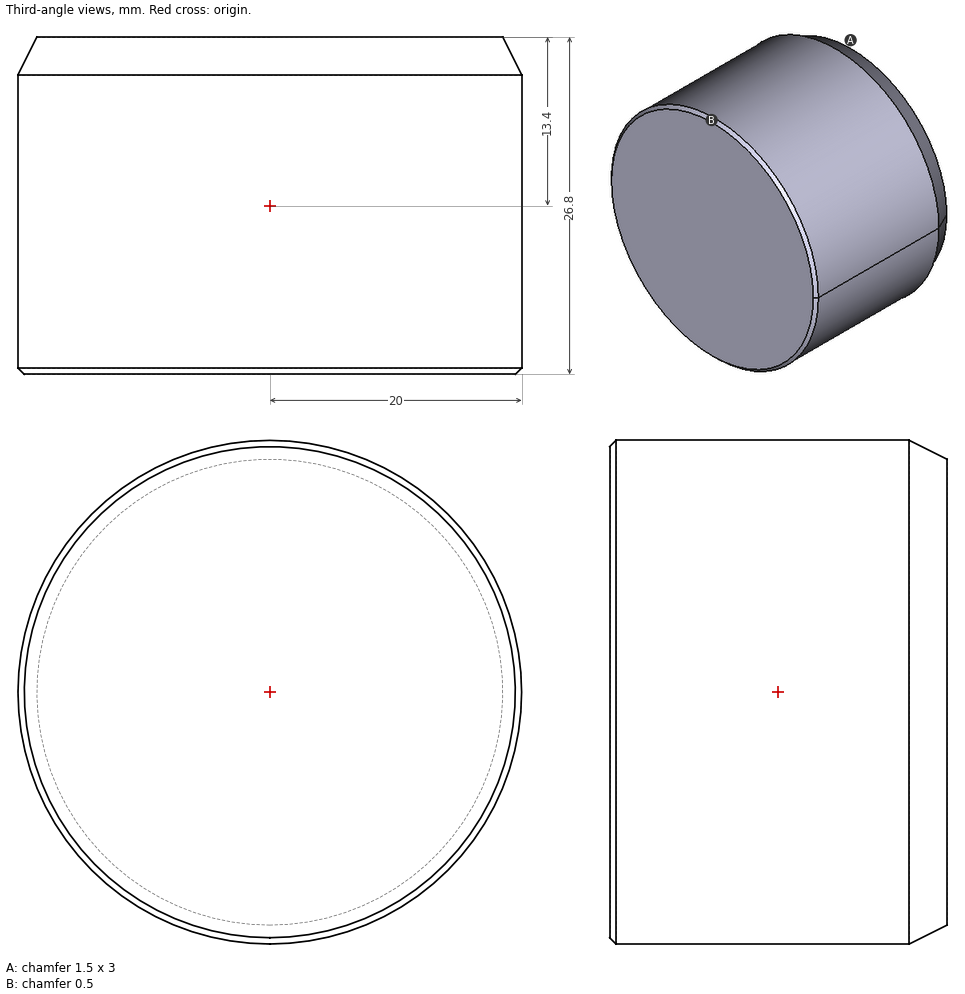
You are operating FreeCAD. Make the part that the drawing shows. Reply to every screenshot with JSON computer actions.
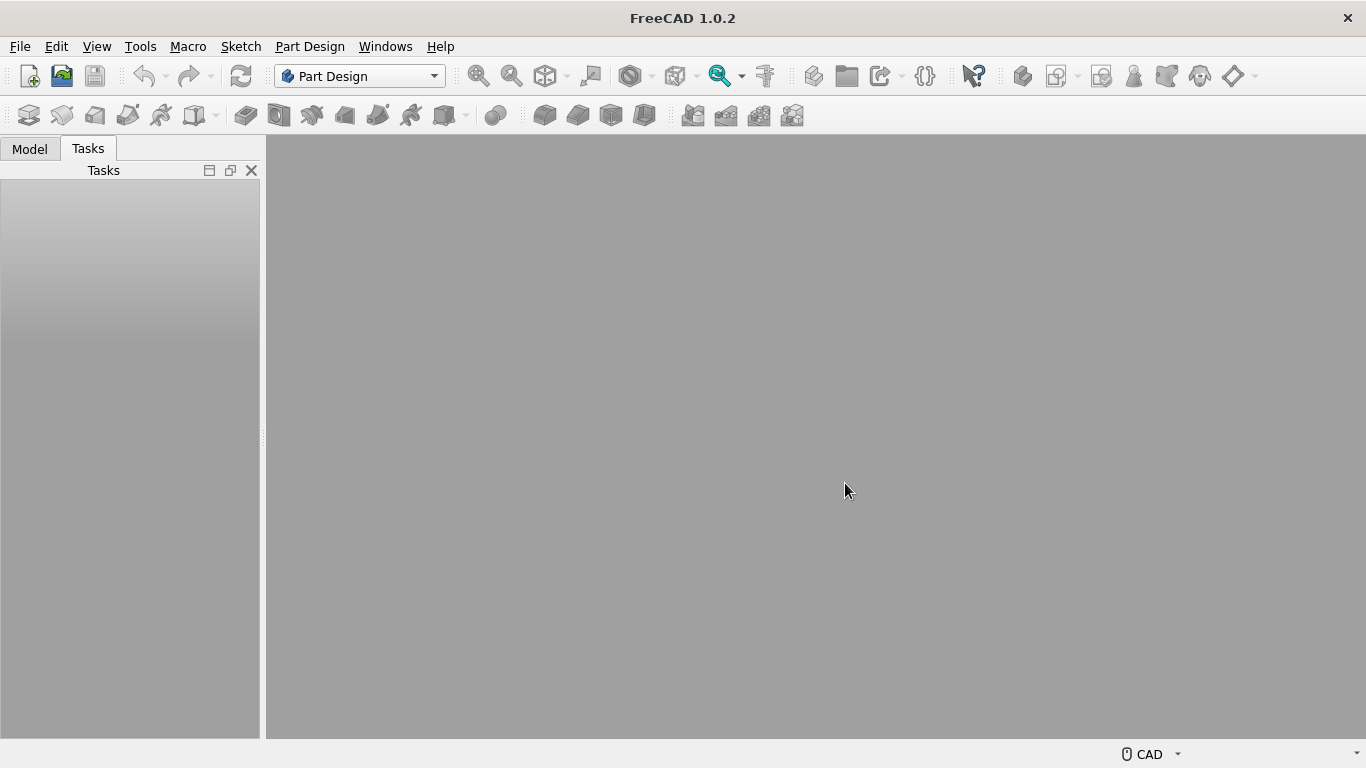
{"action": "left_click", "coordinate": [29, 76]}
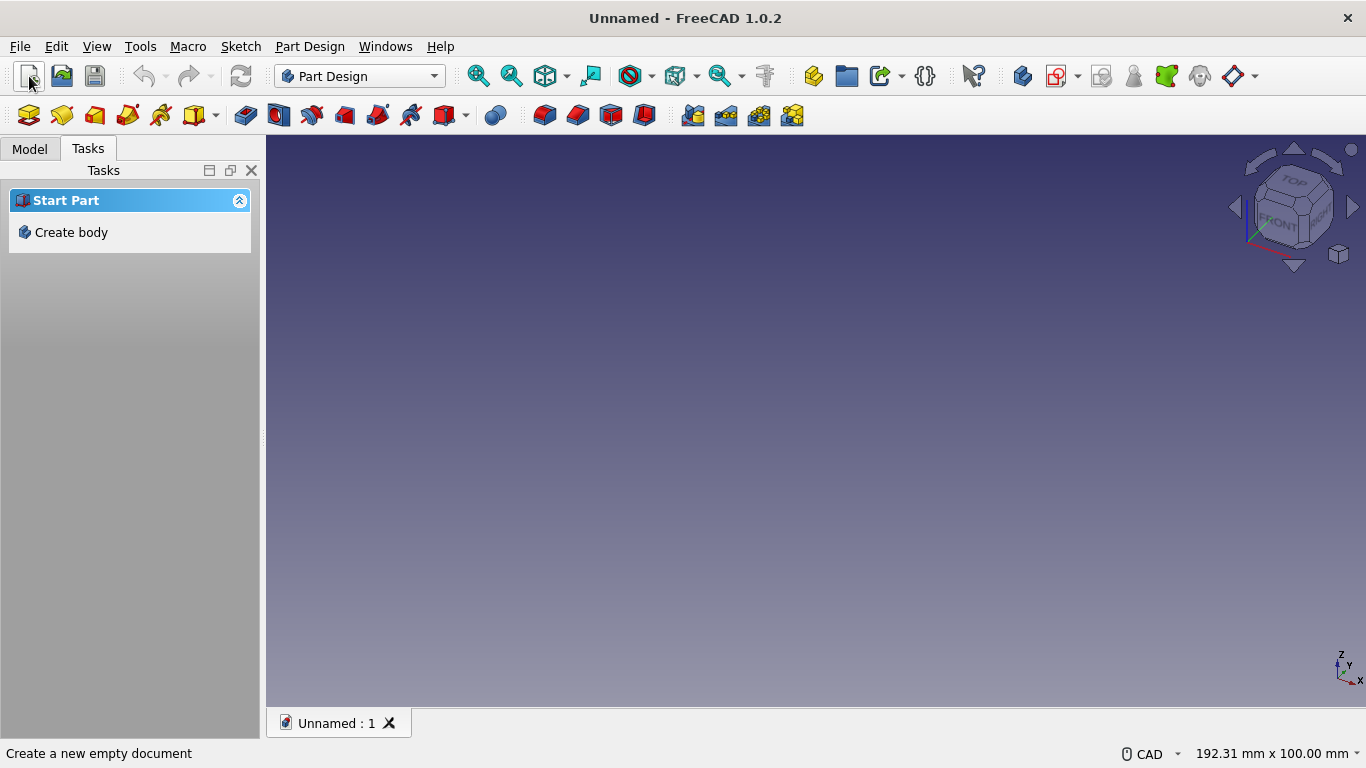
{"action": "left_click", "coordinate": [1056, 76]}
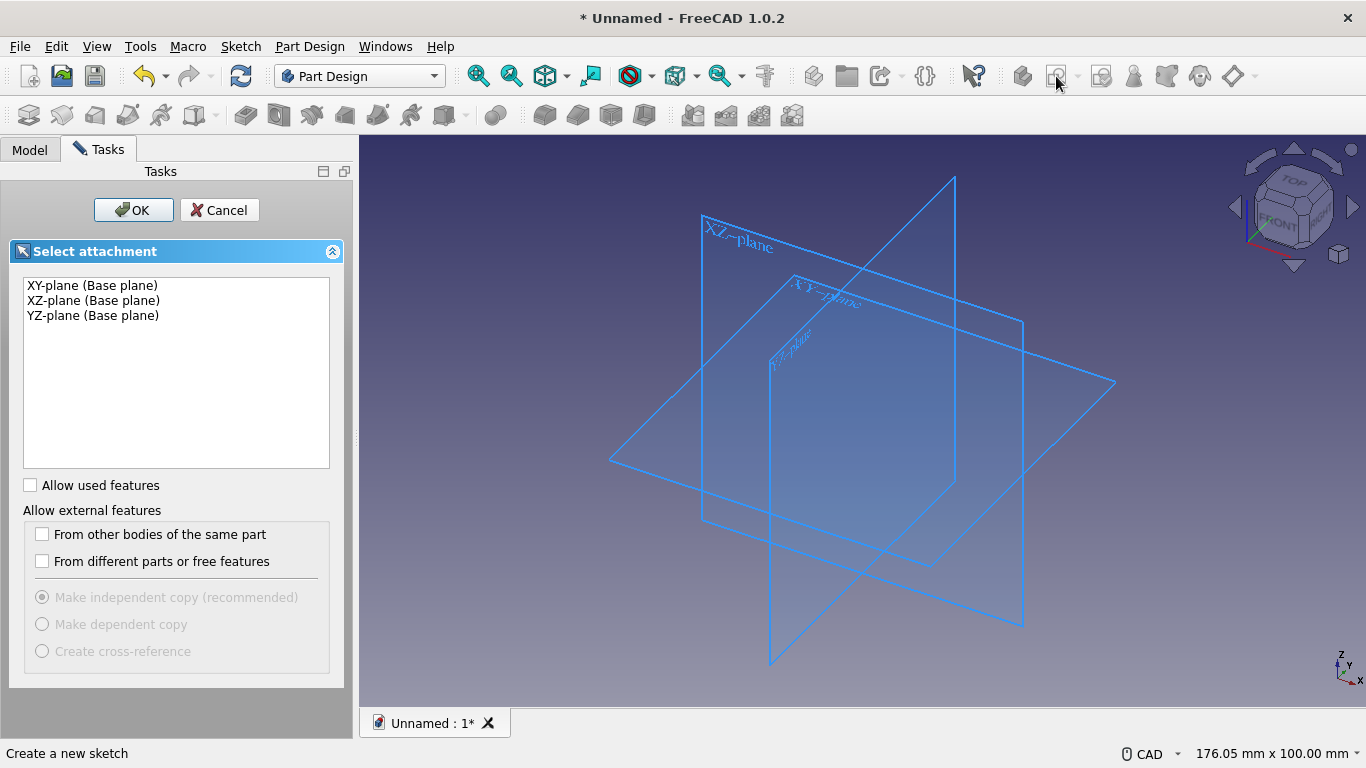
{"action": "left_click", "coordinate": [84, 286]}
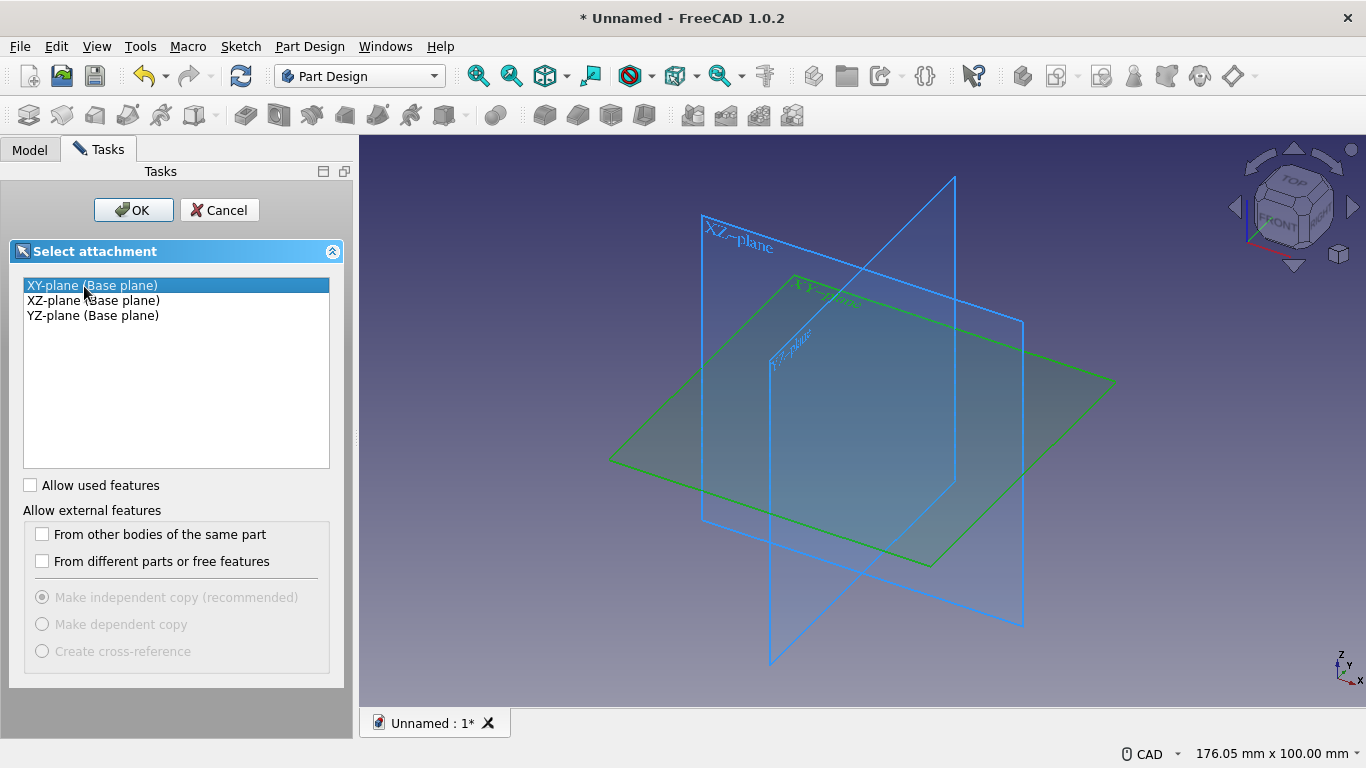
{"action": "left_click", "coordinate": [134, 210]}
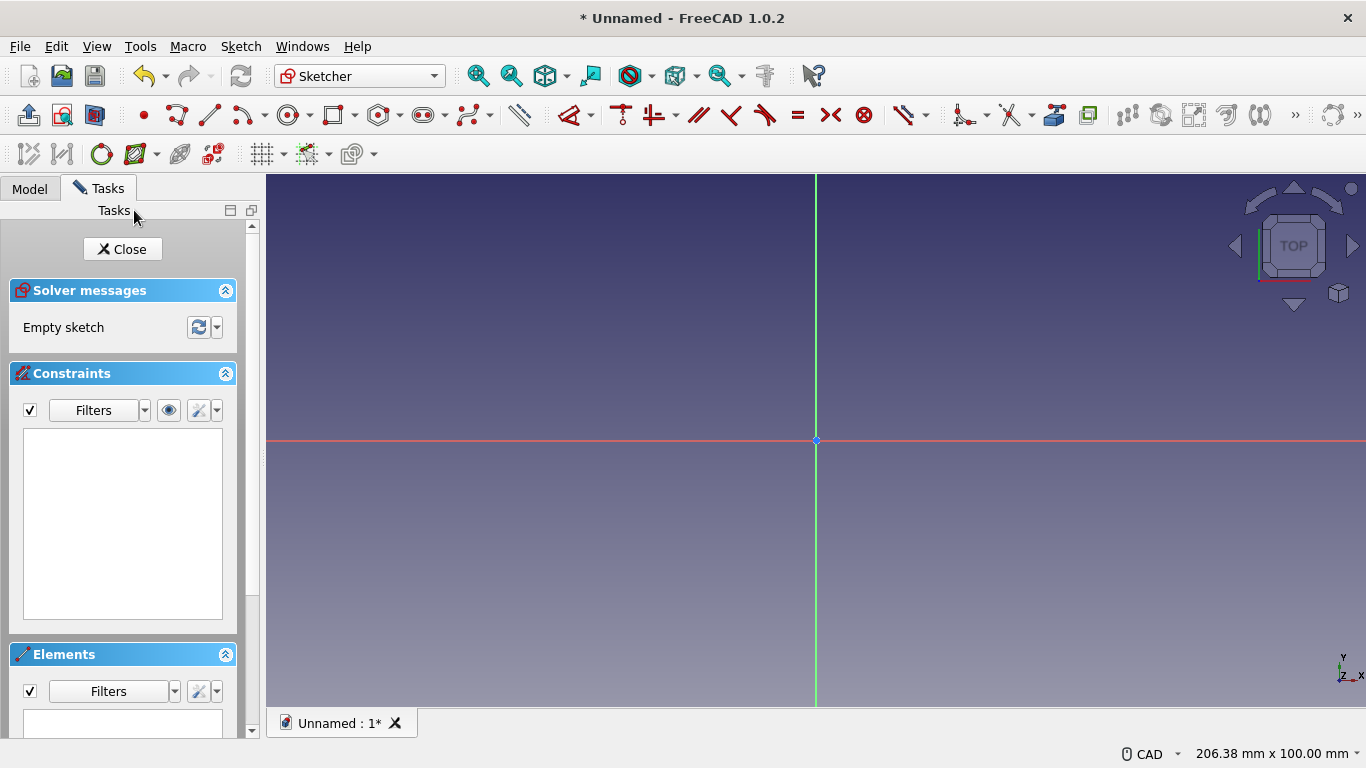
{"action": "scroll", "coordinate": [969, 440], "scroll_direction": "up", "scroll_amount": 4}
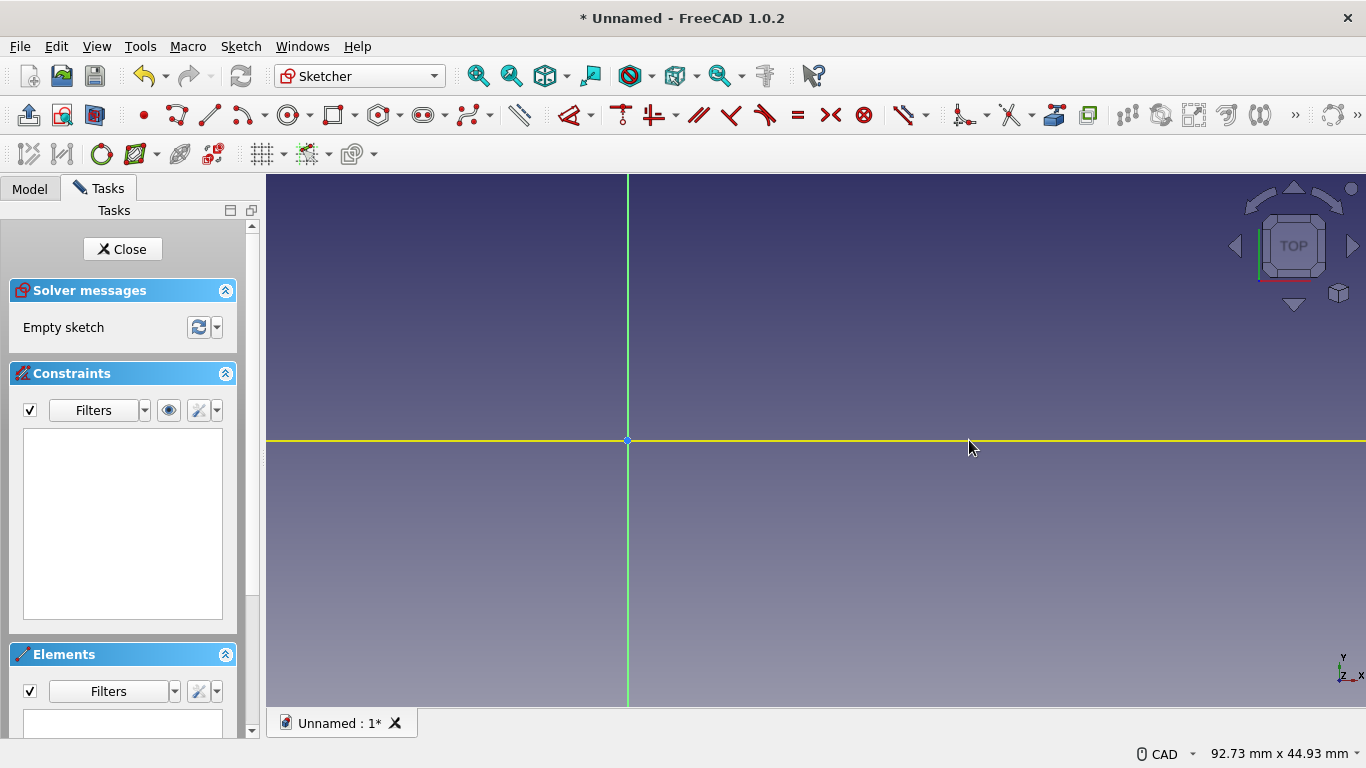
{"action": "key", "text": "g r"}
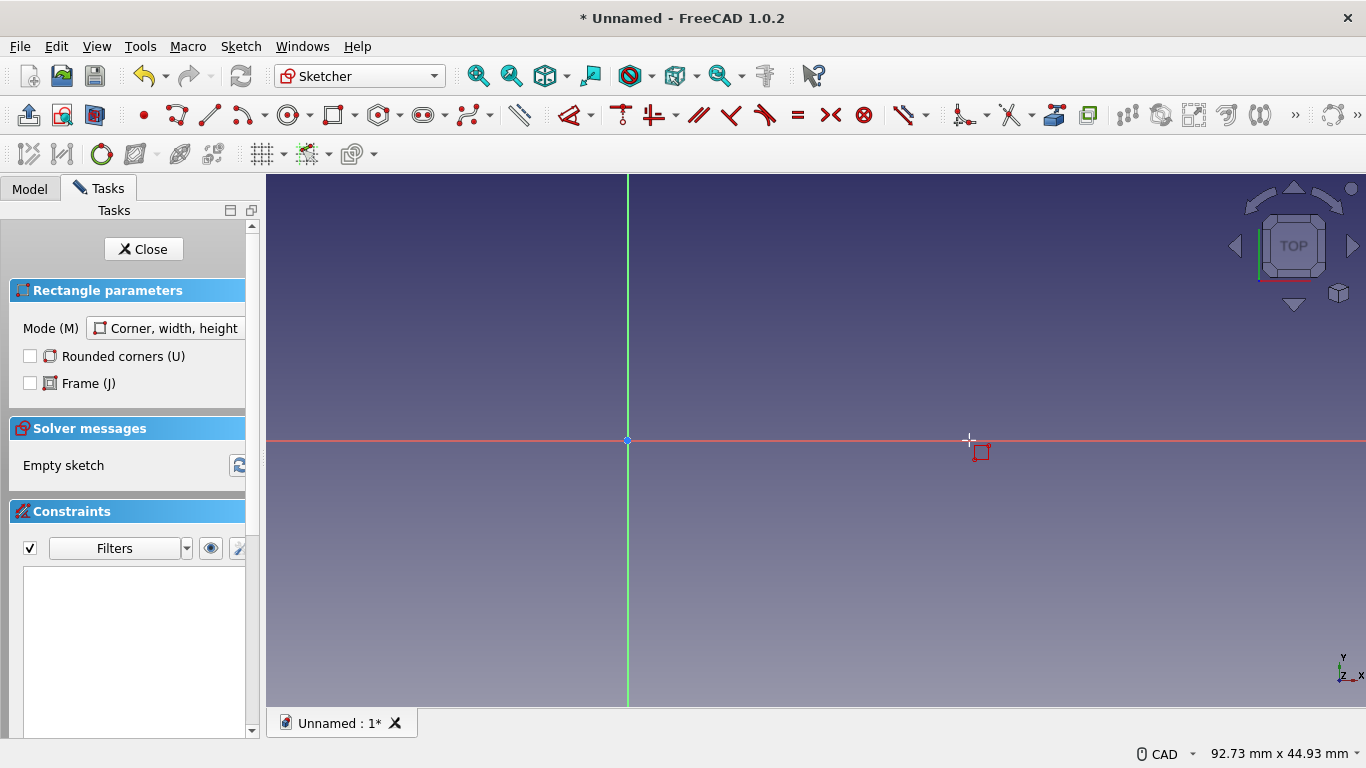
{"action": "left_click", "coordinate": [628, 282]}
{"action": "left_click", "coordinate": [865, 599]}
{"action": "key", "text": "Escape"}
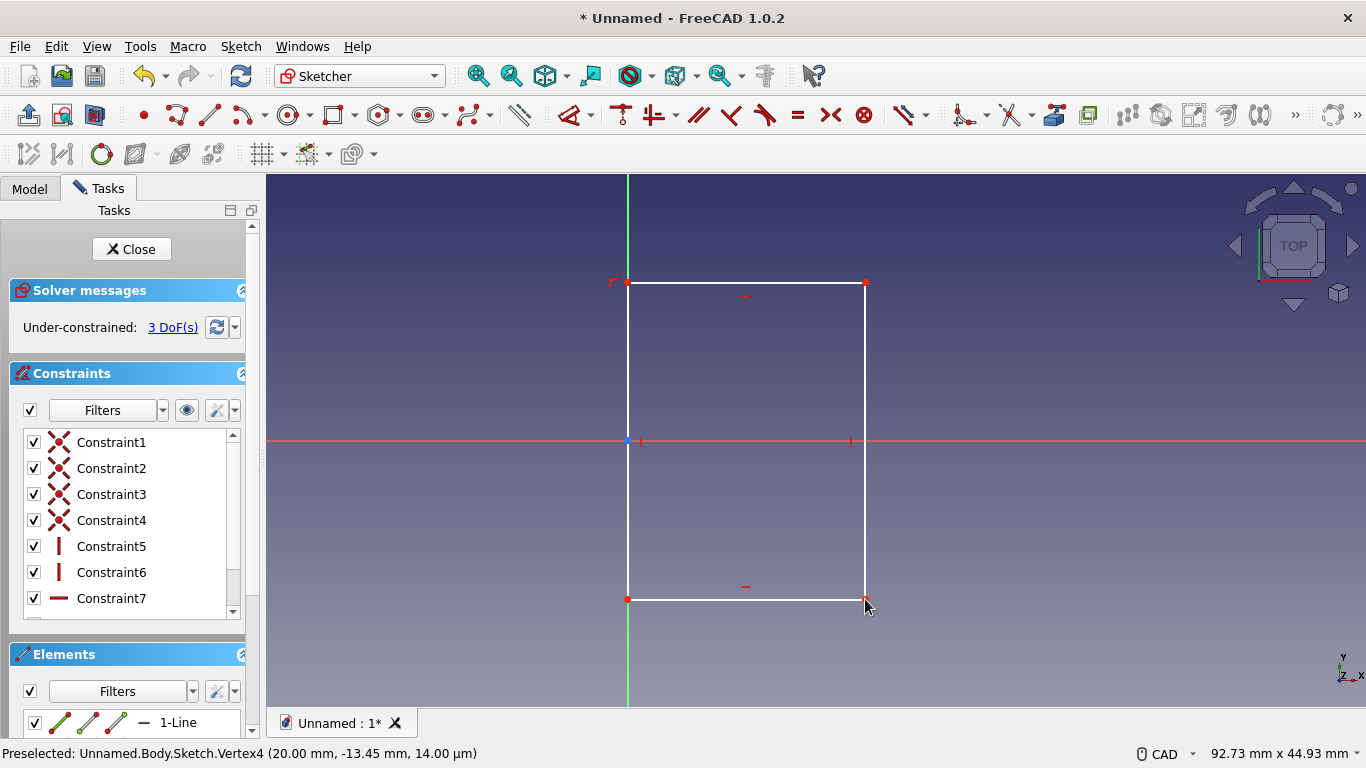
{"action": "left_click", "coordinate": [699, 600]}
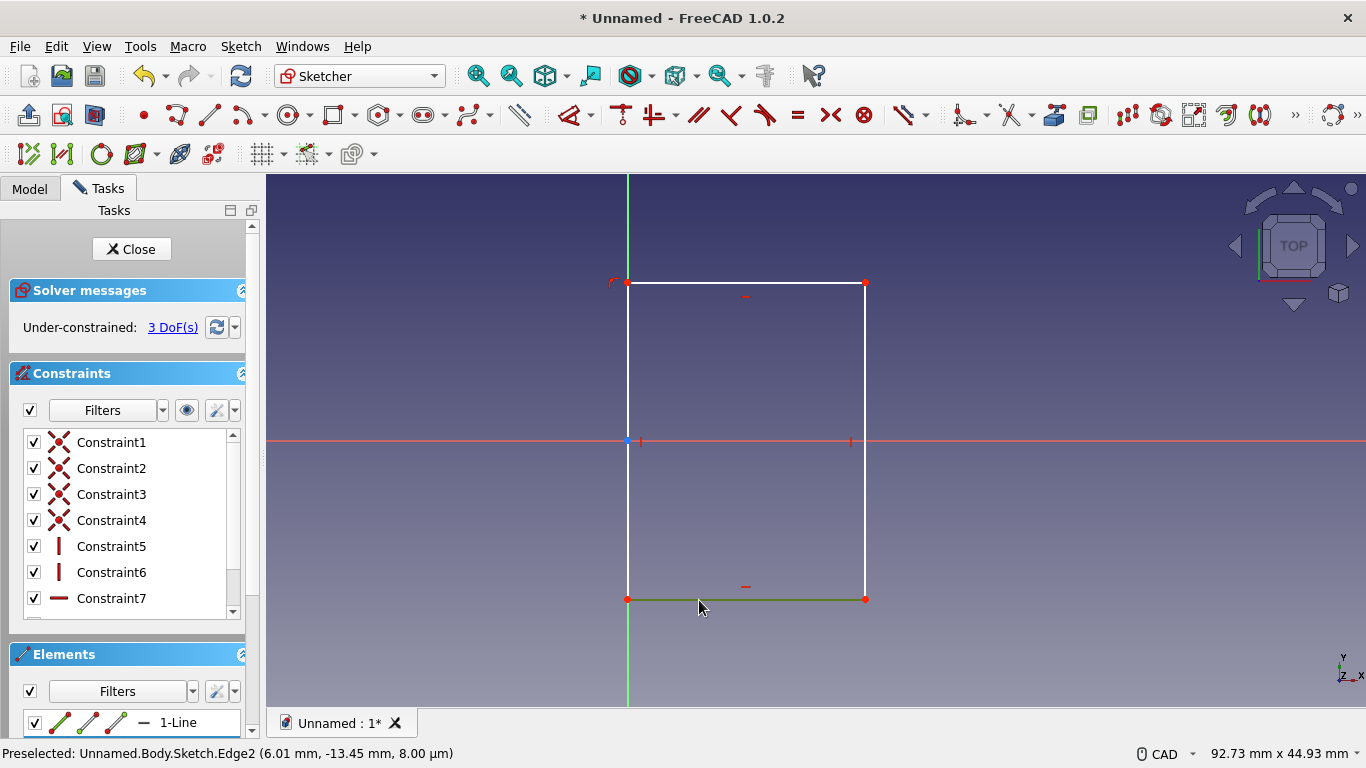
{"action": "left_click", "coordinate": [590, 116]}